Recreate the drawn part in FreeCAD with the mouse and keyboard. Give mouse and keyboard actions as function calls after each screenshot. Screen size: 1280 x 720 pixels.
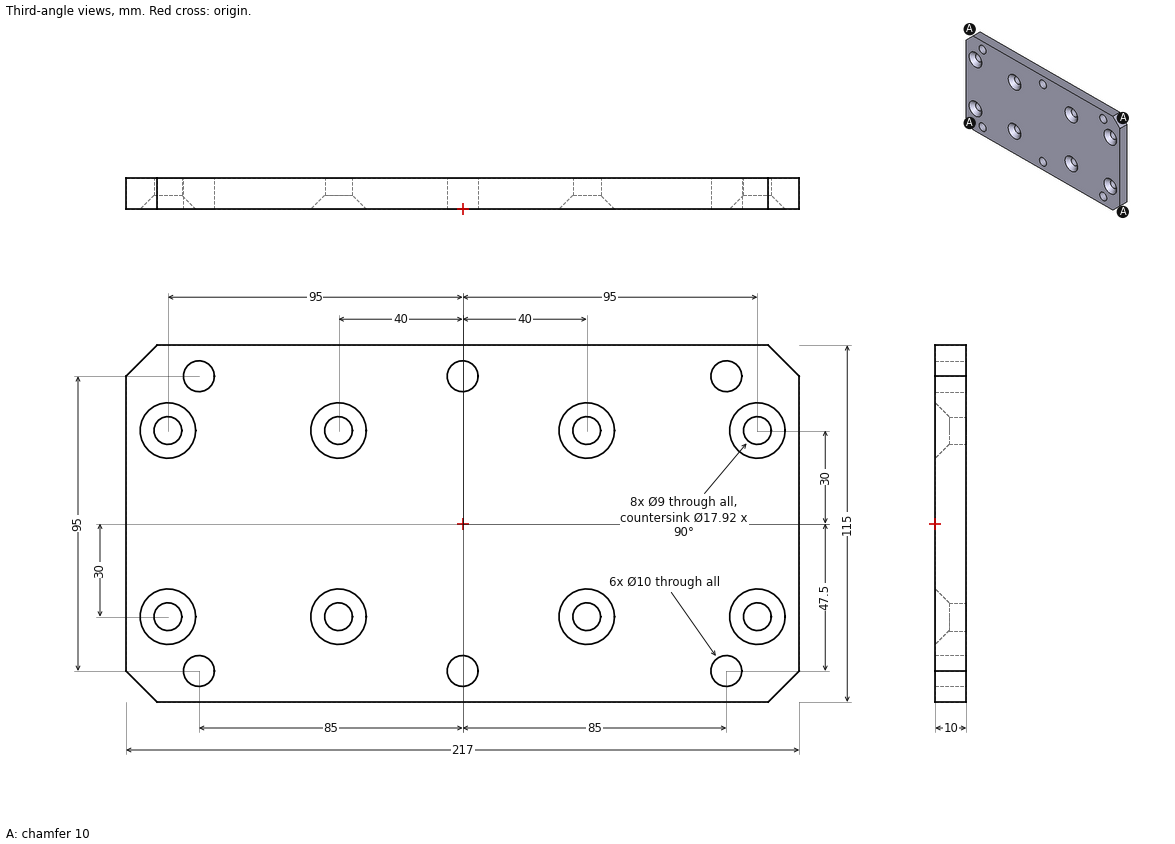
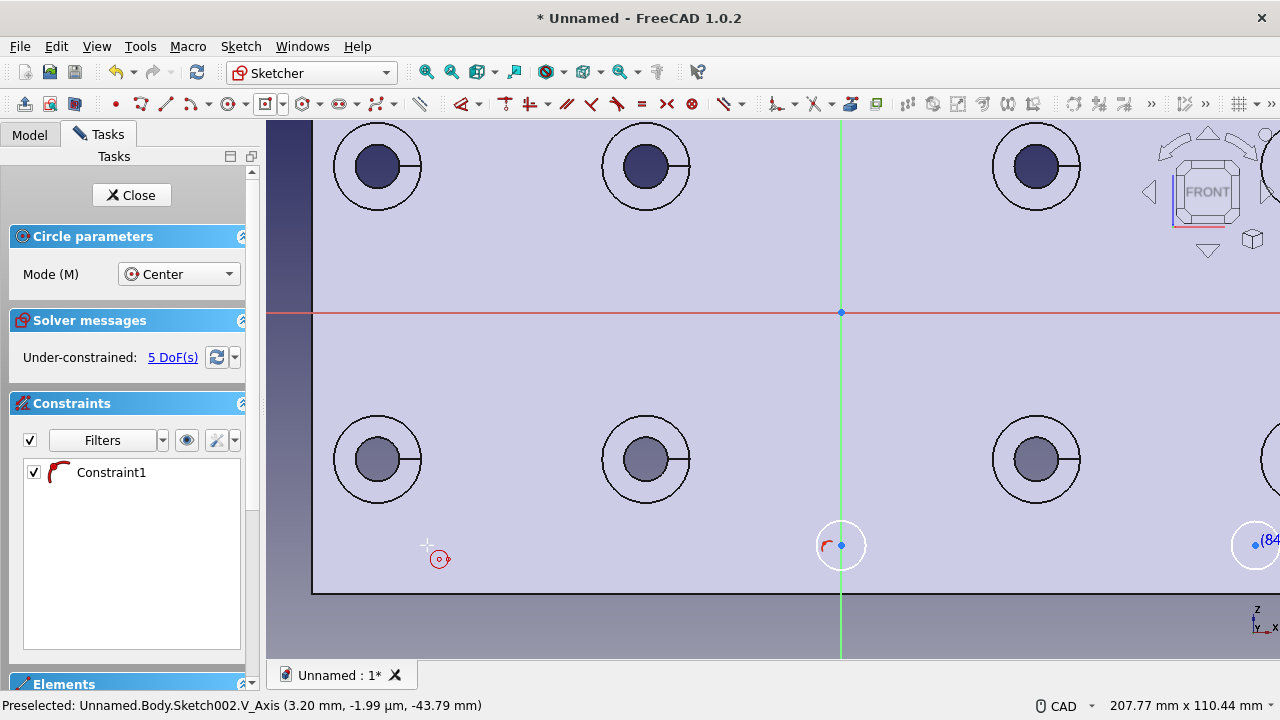
click(426, 545)
click(444, 527)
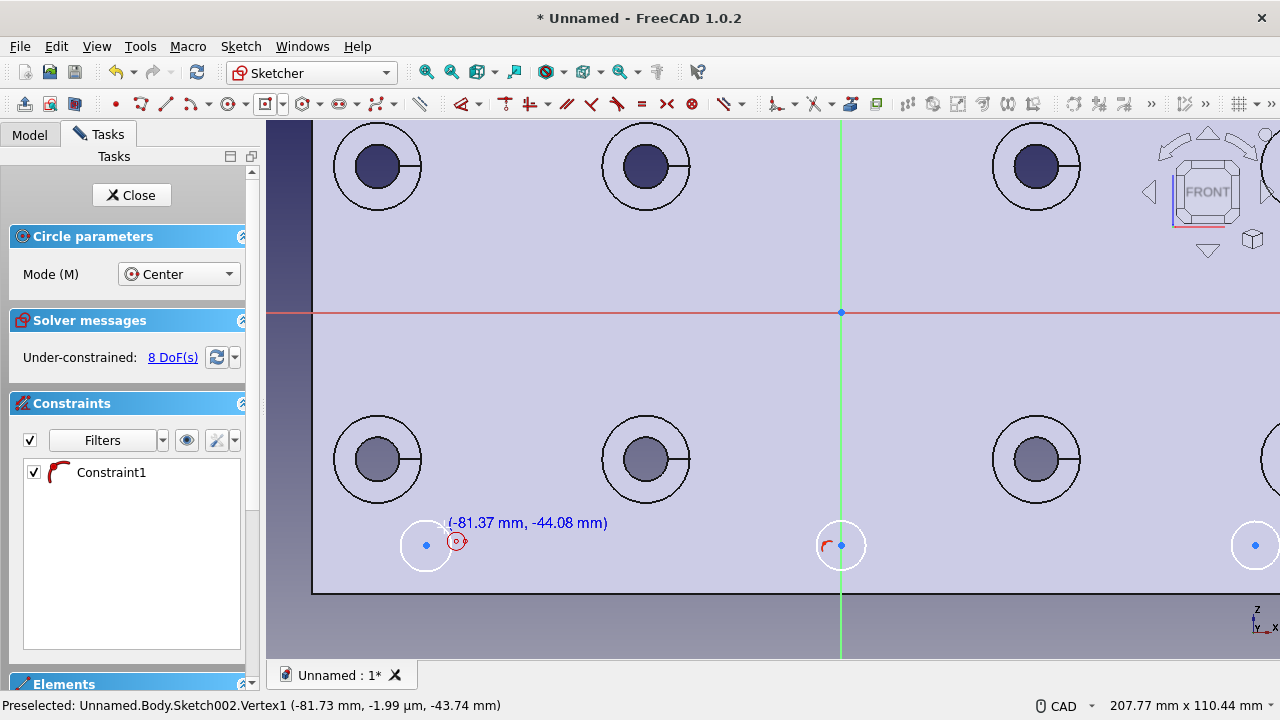
scroll(427, 545, down, 2)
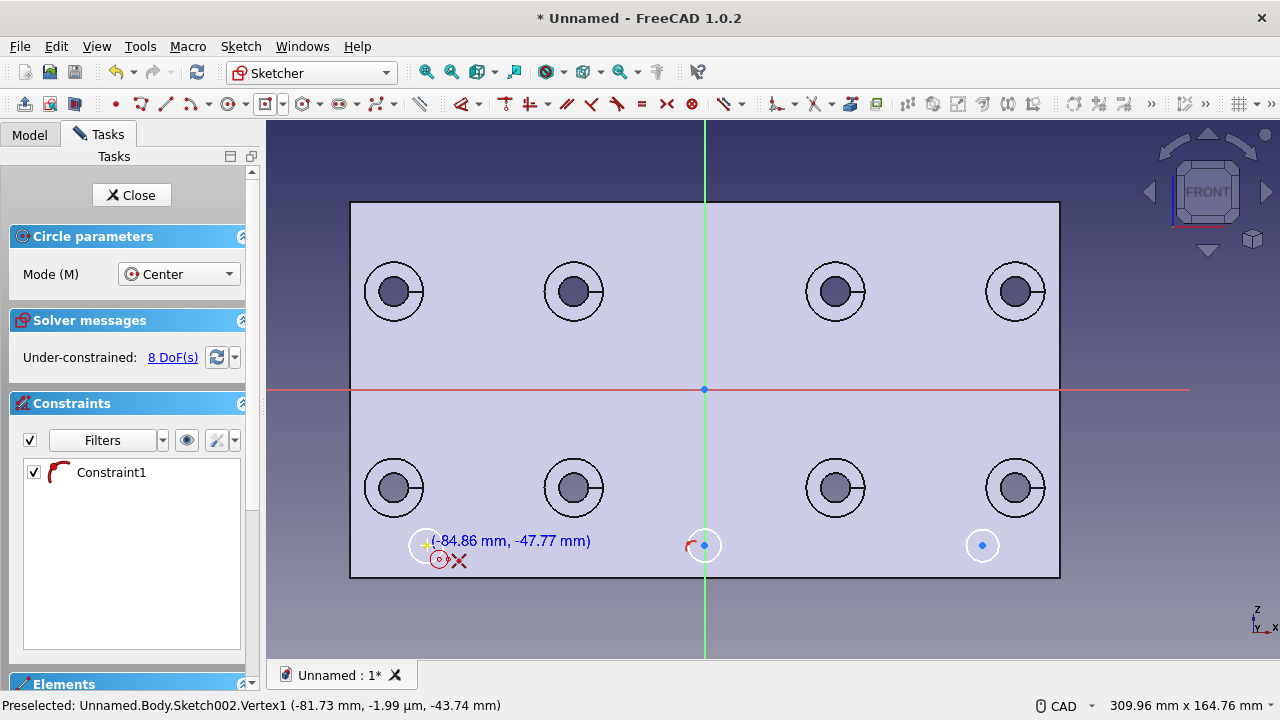
scroll(427, 234, up, 2)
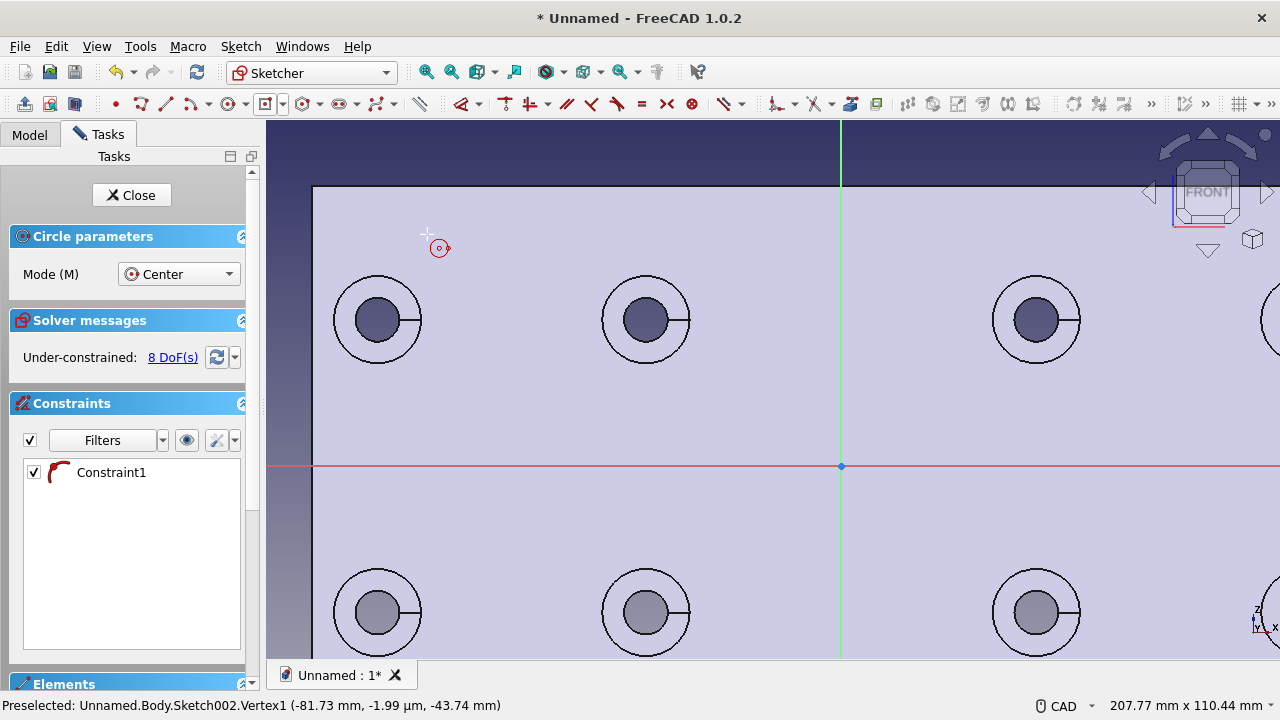
click(426, 234)
click(444, 217)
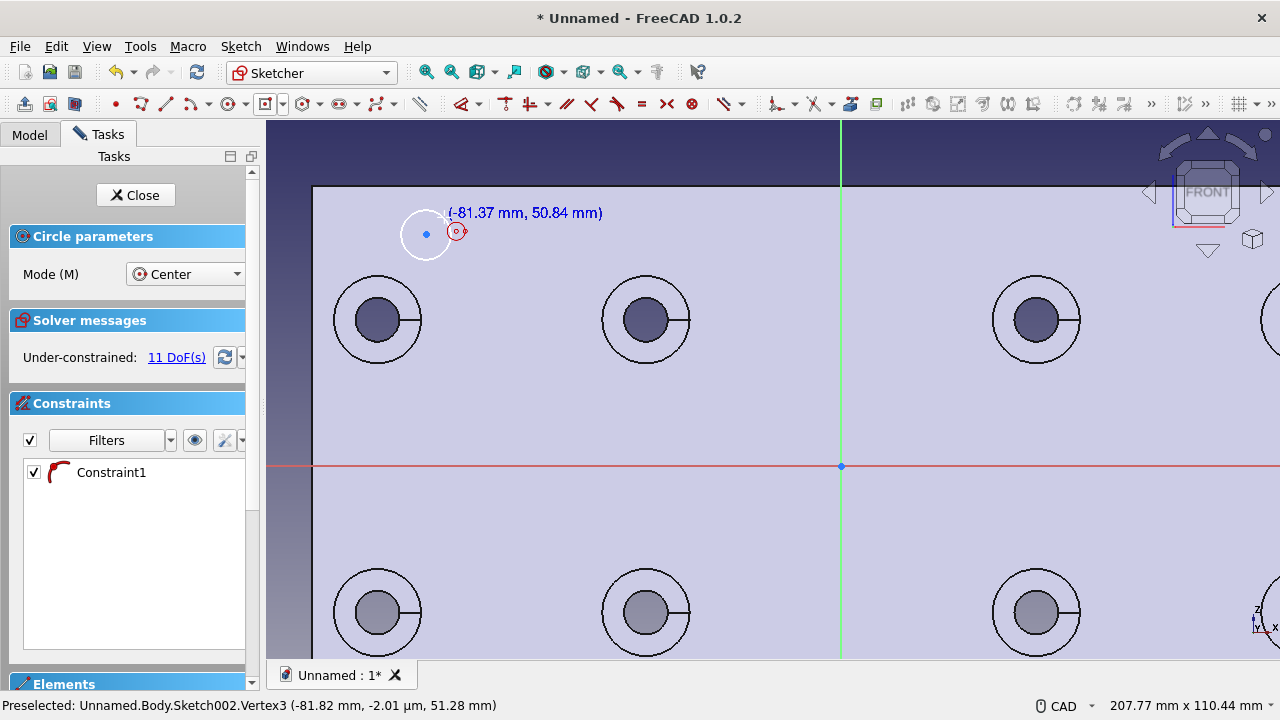
click(841, 234)
click(858, 217)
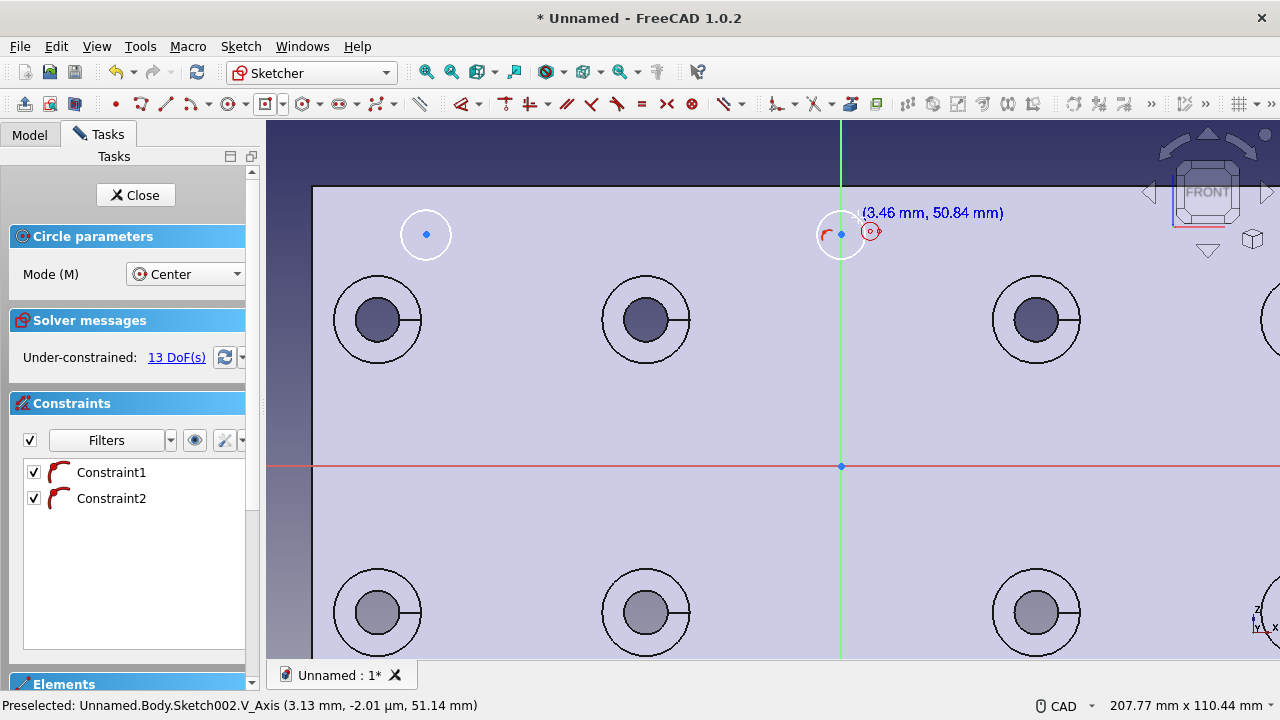
scroll(427, 234, down, 2)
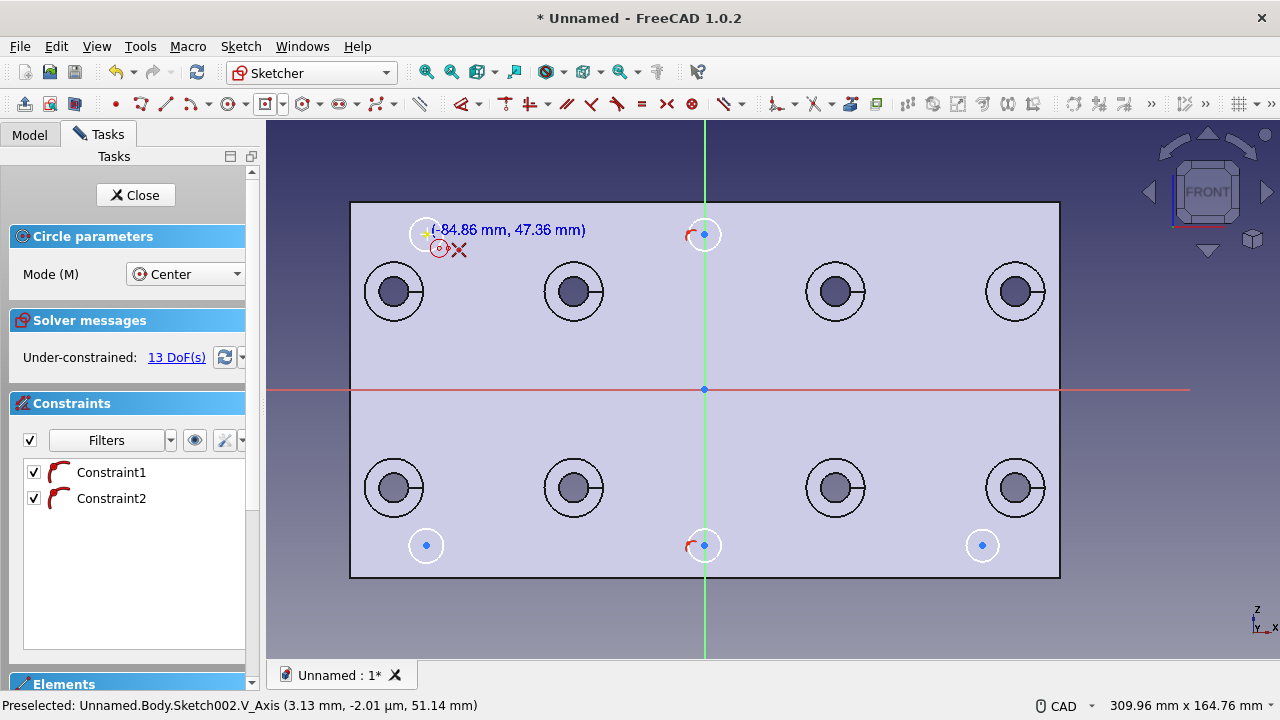
scroll(983, 234, up, 2)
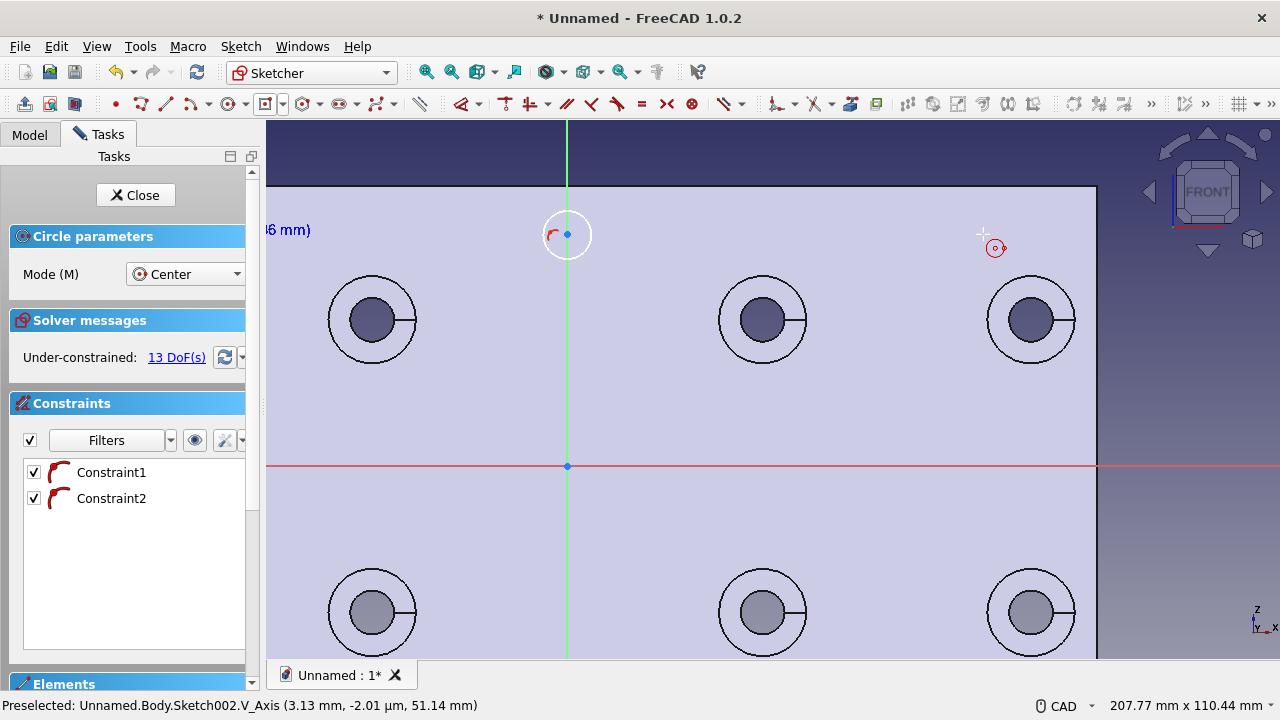
click(982, 234)
click(999, 217)
key(Escape)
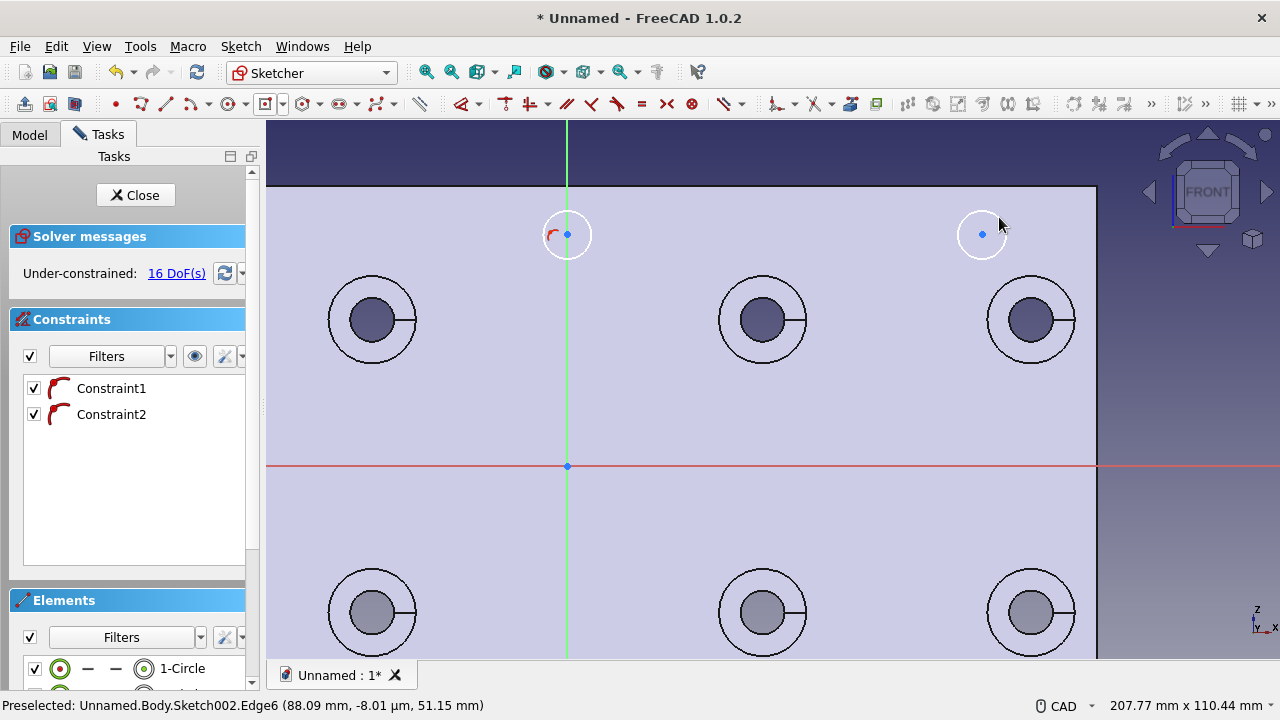
scroll(983, 234, down, 2)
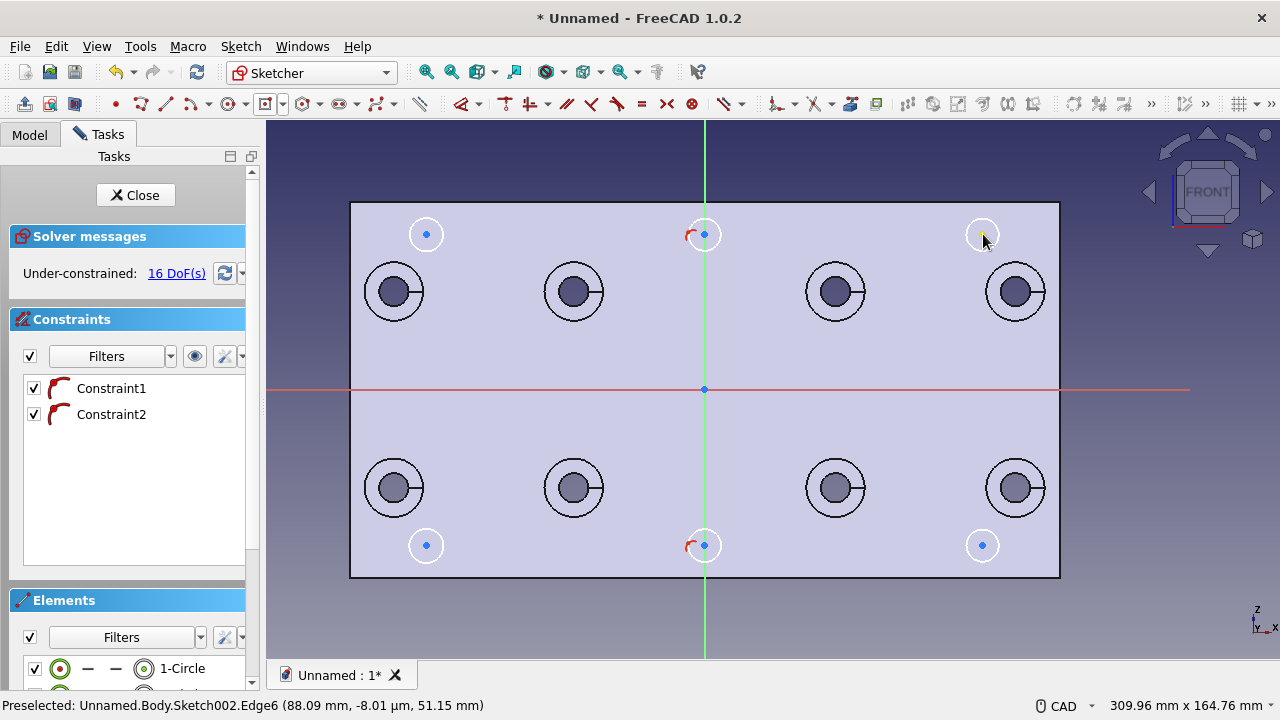
click(994, 534)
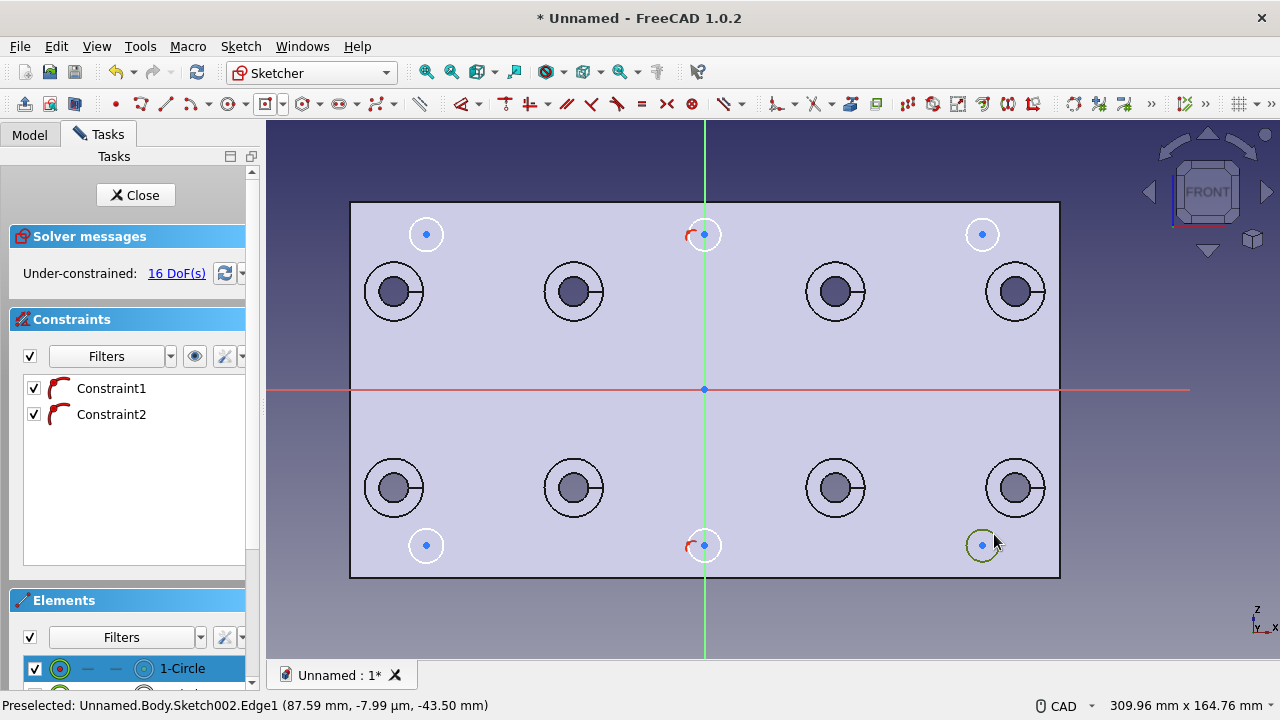
click(716, 534)